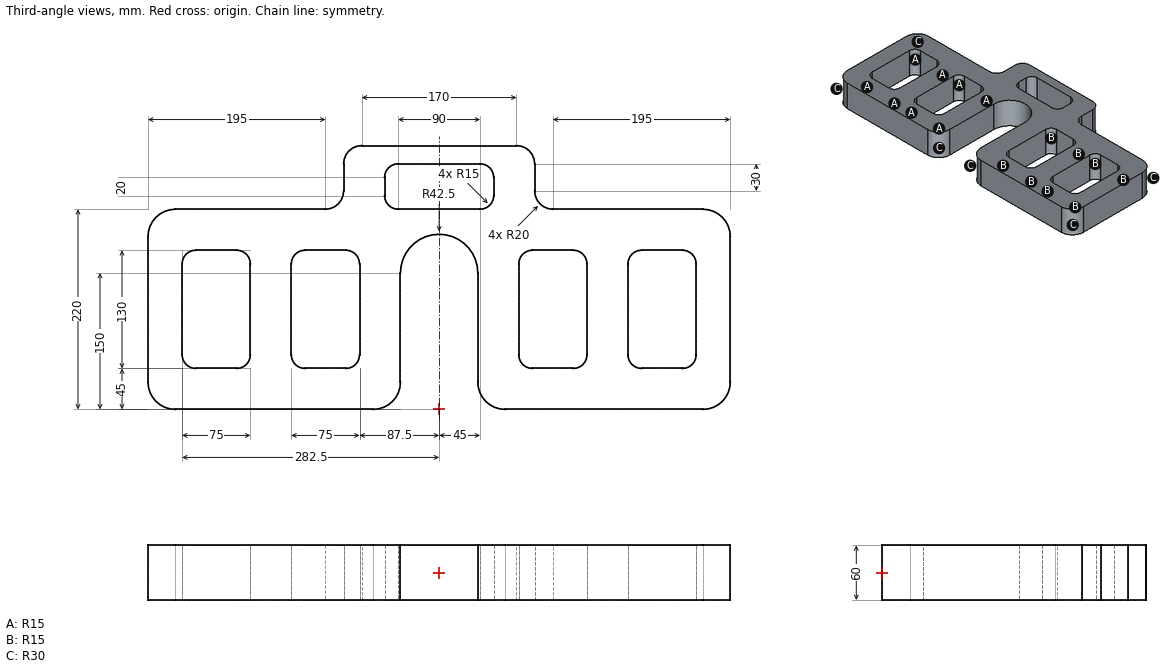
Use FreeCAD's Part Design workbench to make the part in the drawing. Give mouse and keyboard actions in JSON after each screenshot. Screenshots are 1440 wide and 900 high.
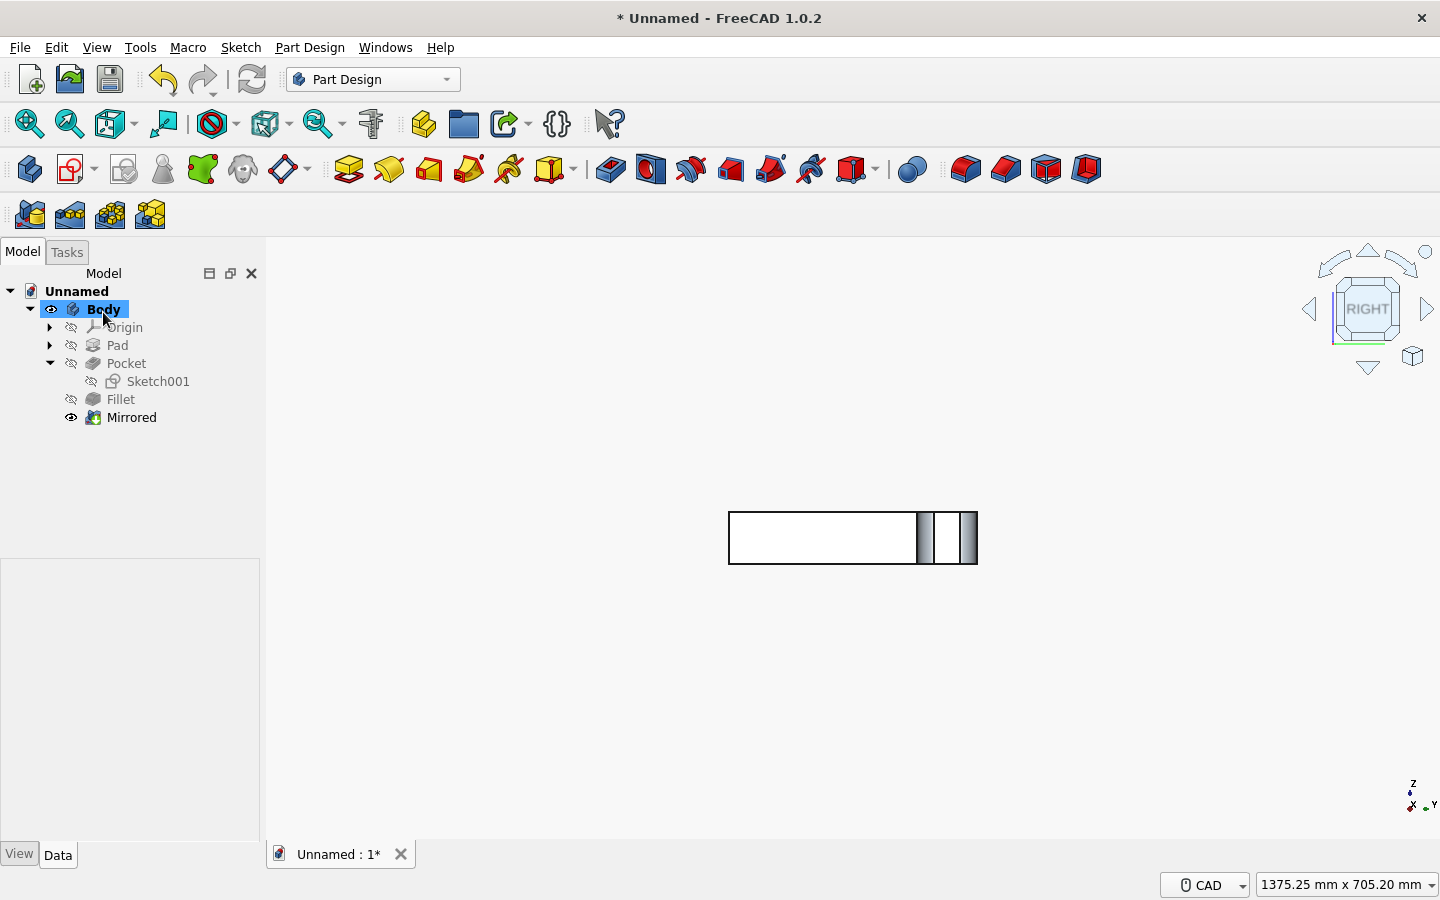
{"action": "key", "text": "5"}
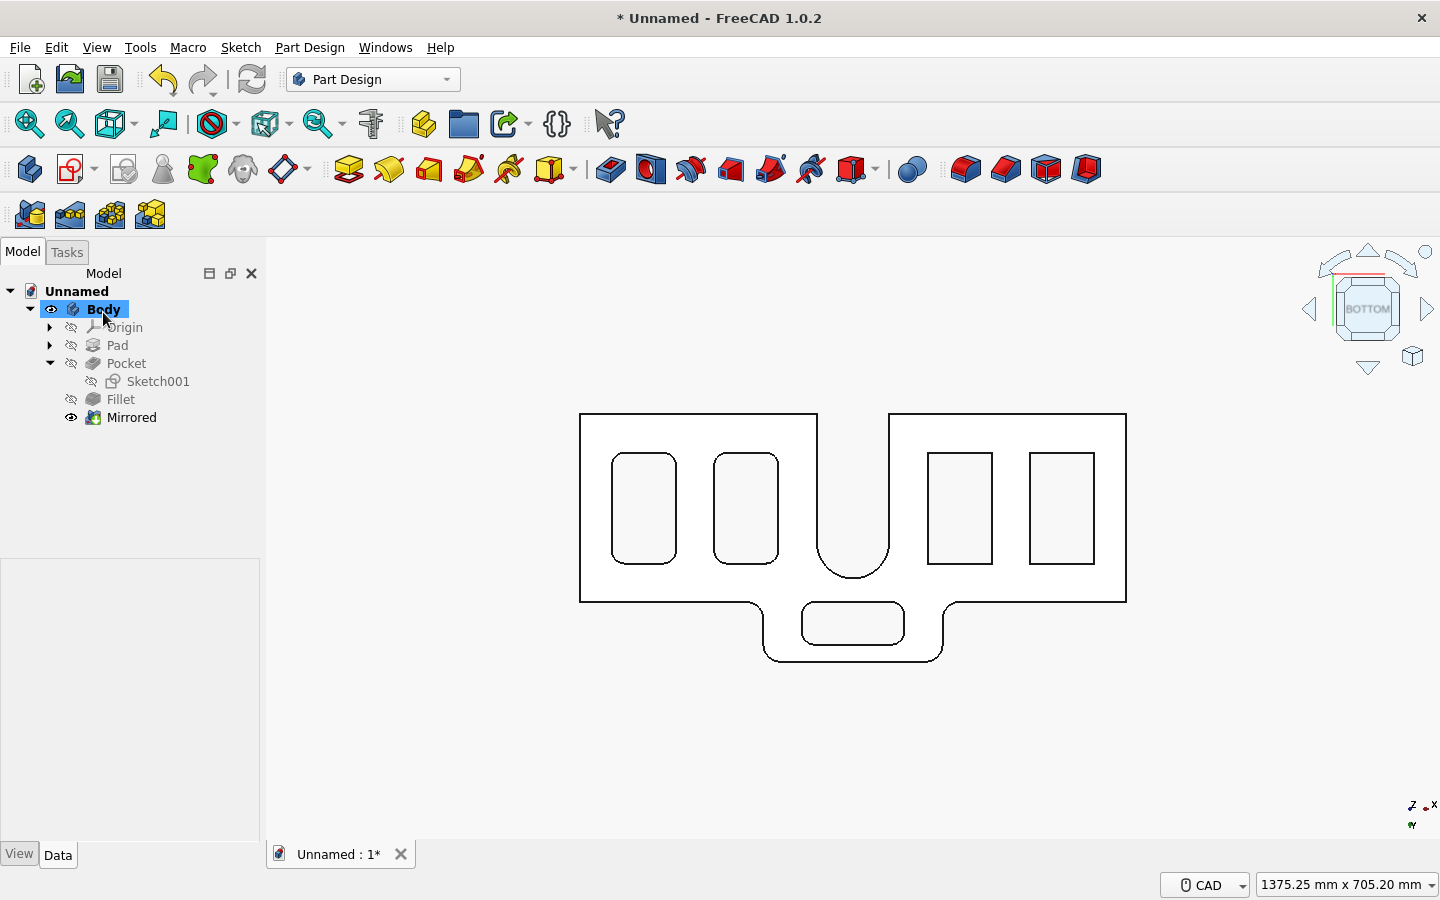
{"action": "key", "text": "4"}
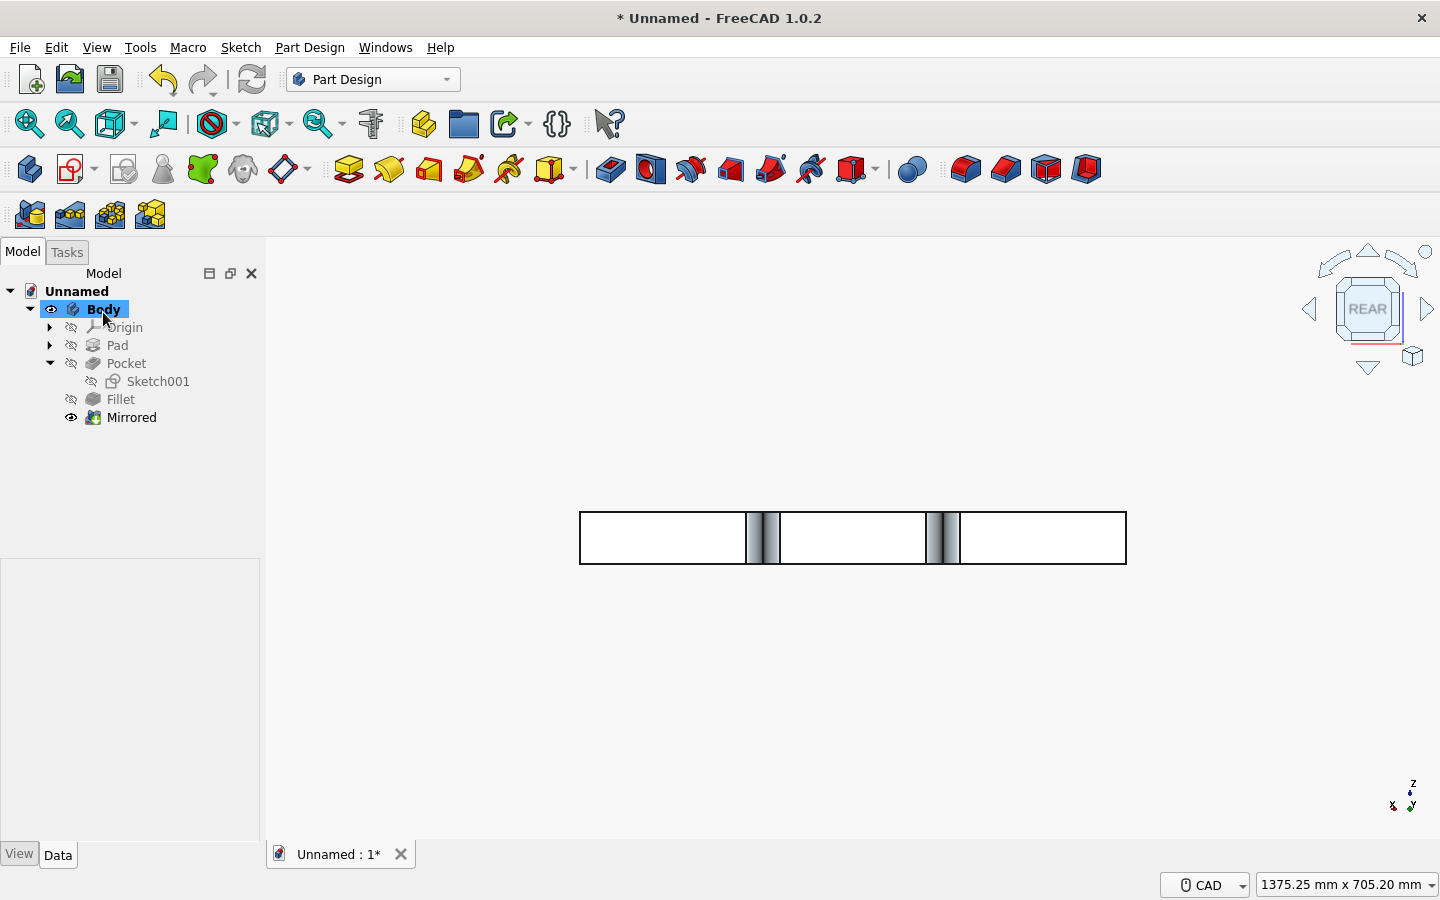
{"action": "key", "text": "6"}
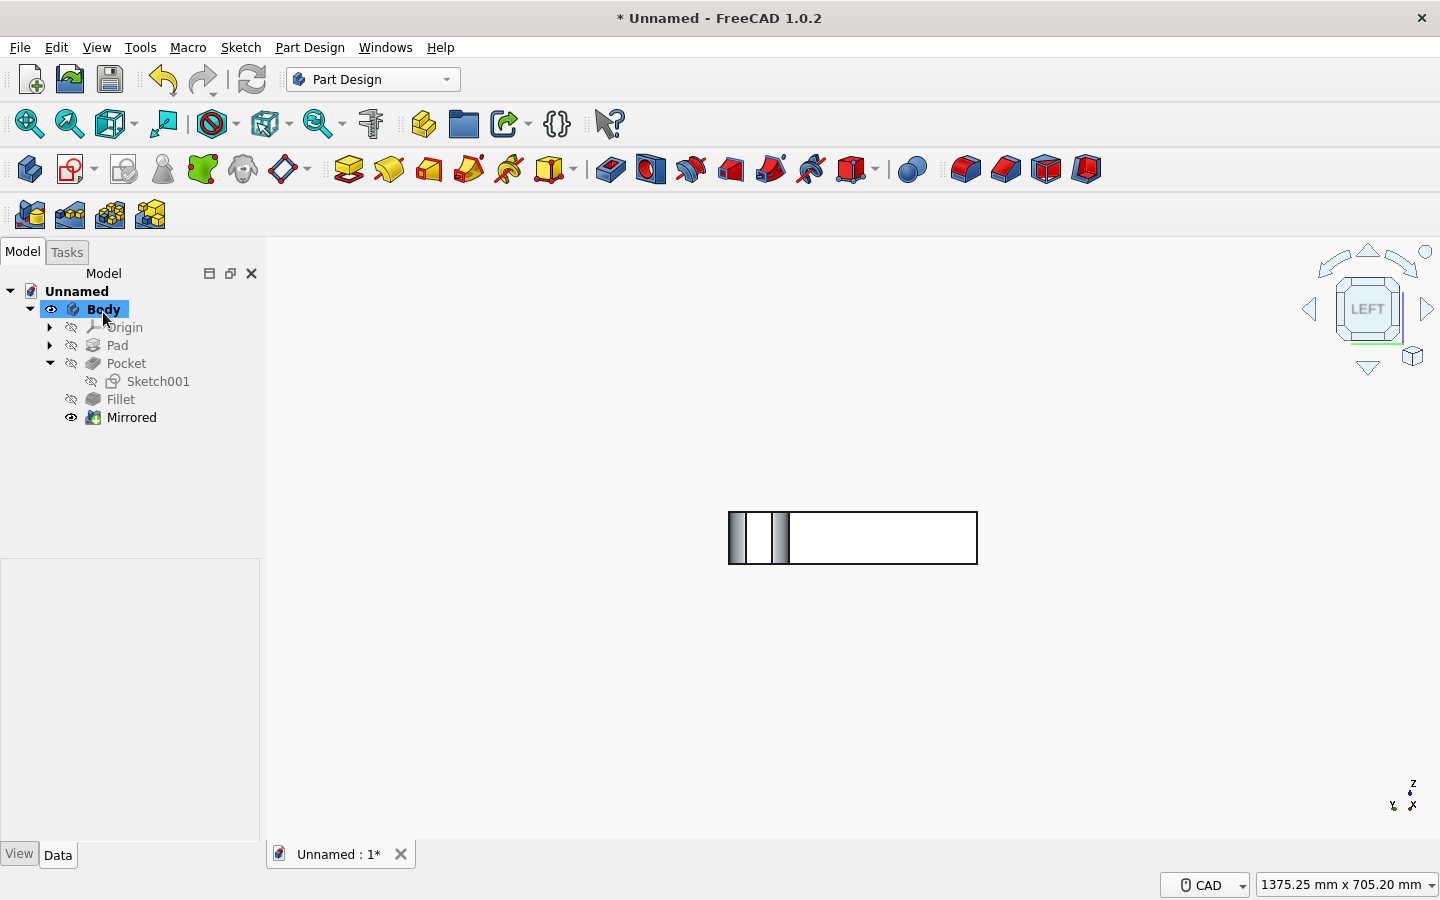
{"action": "left_click", "coordinate": [30, 124]}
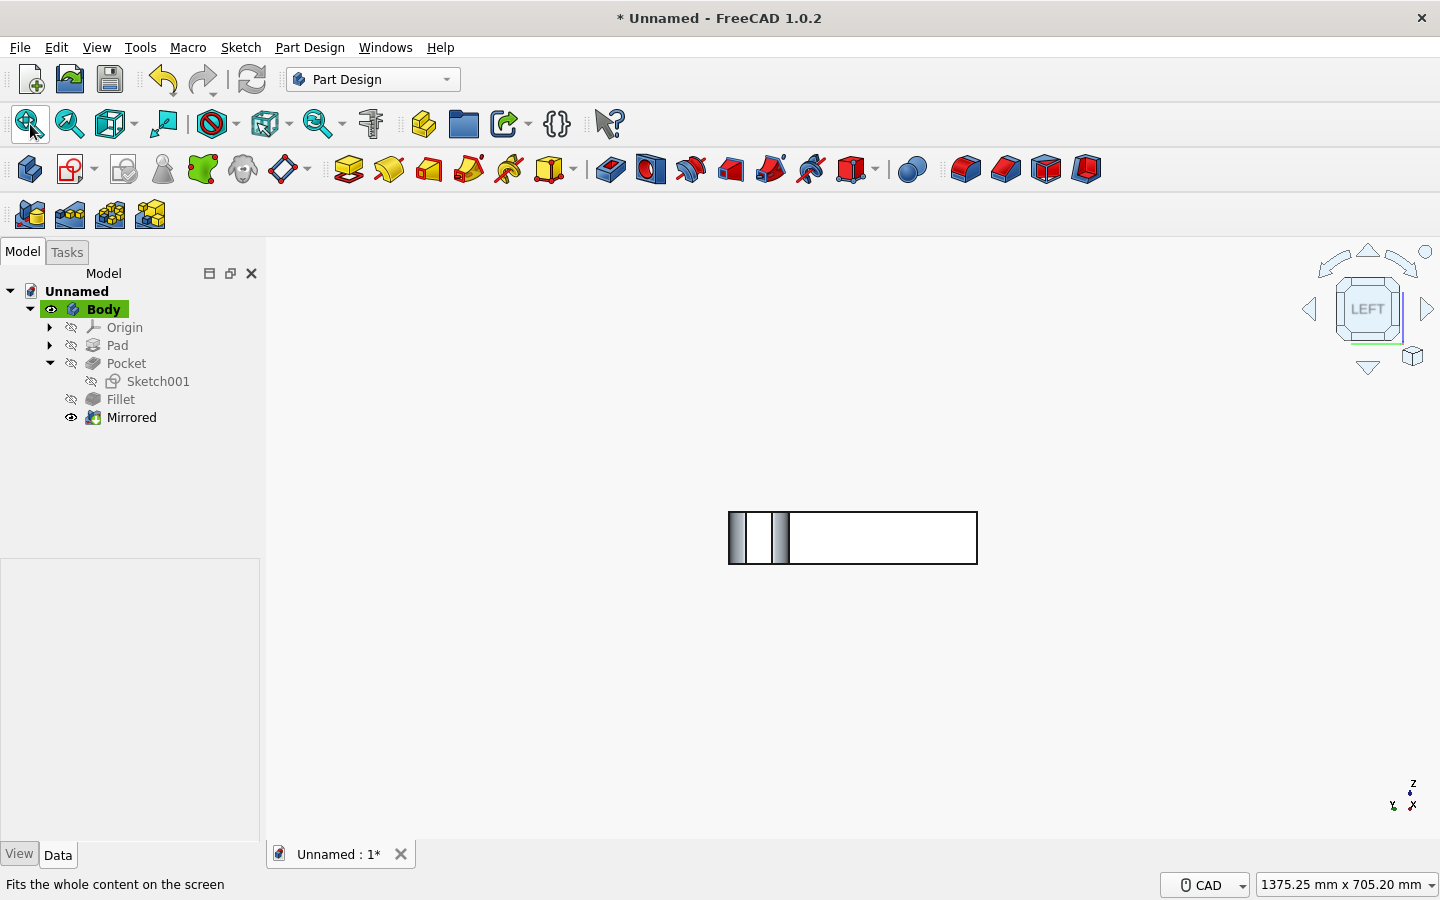
{"action": "key", "text": "v 3"}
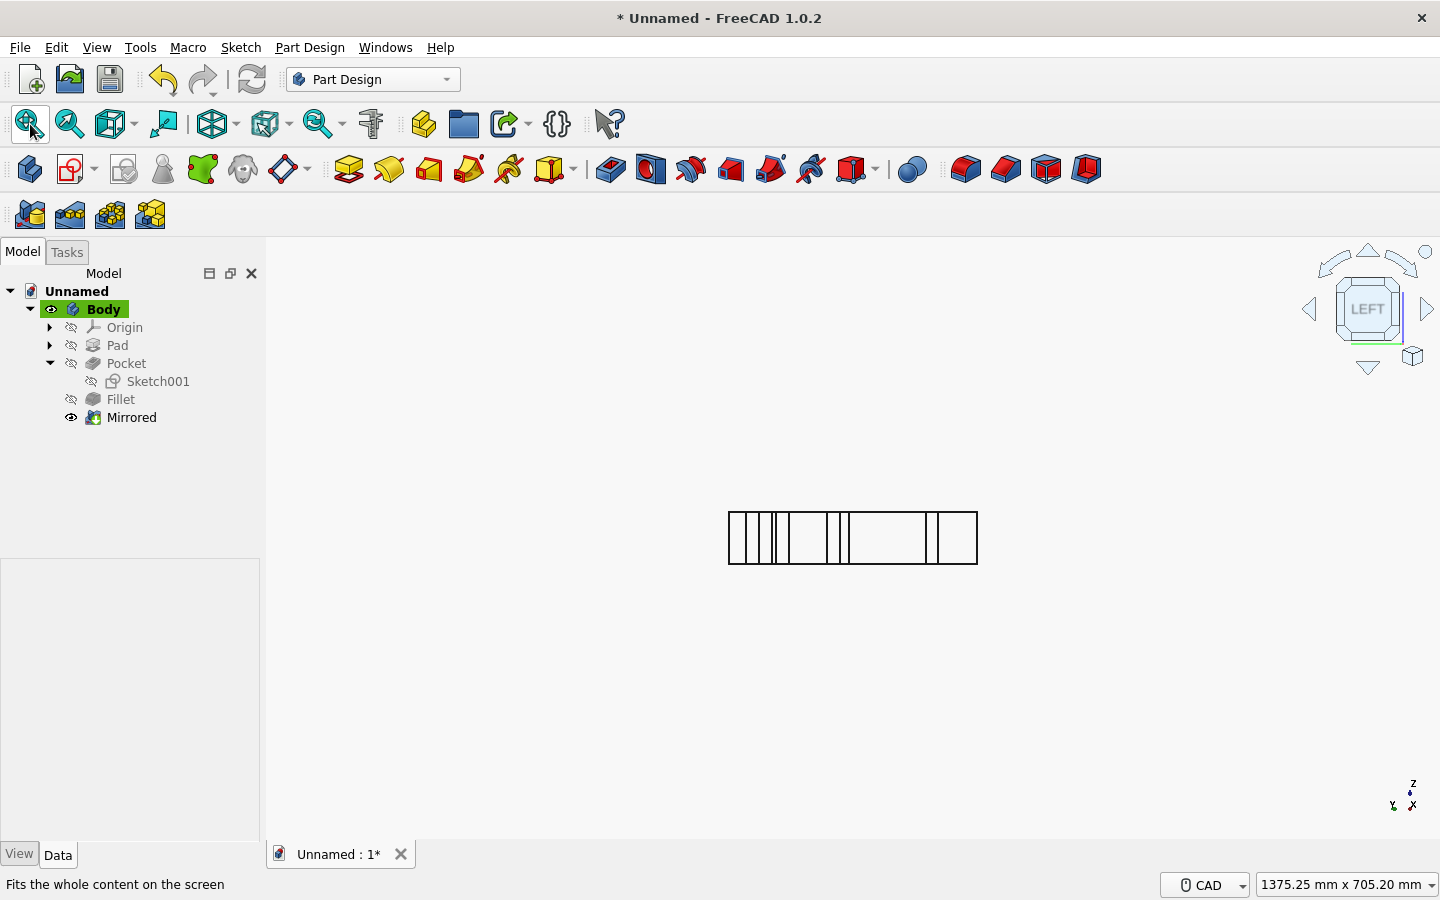
{"action": "key", "text": "0"}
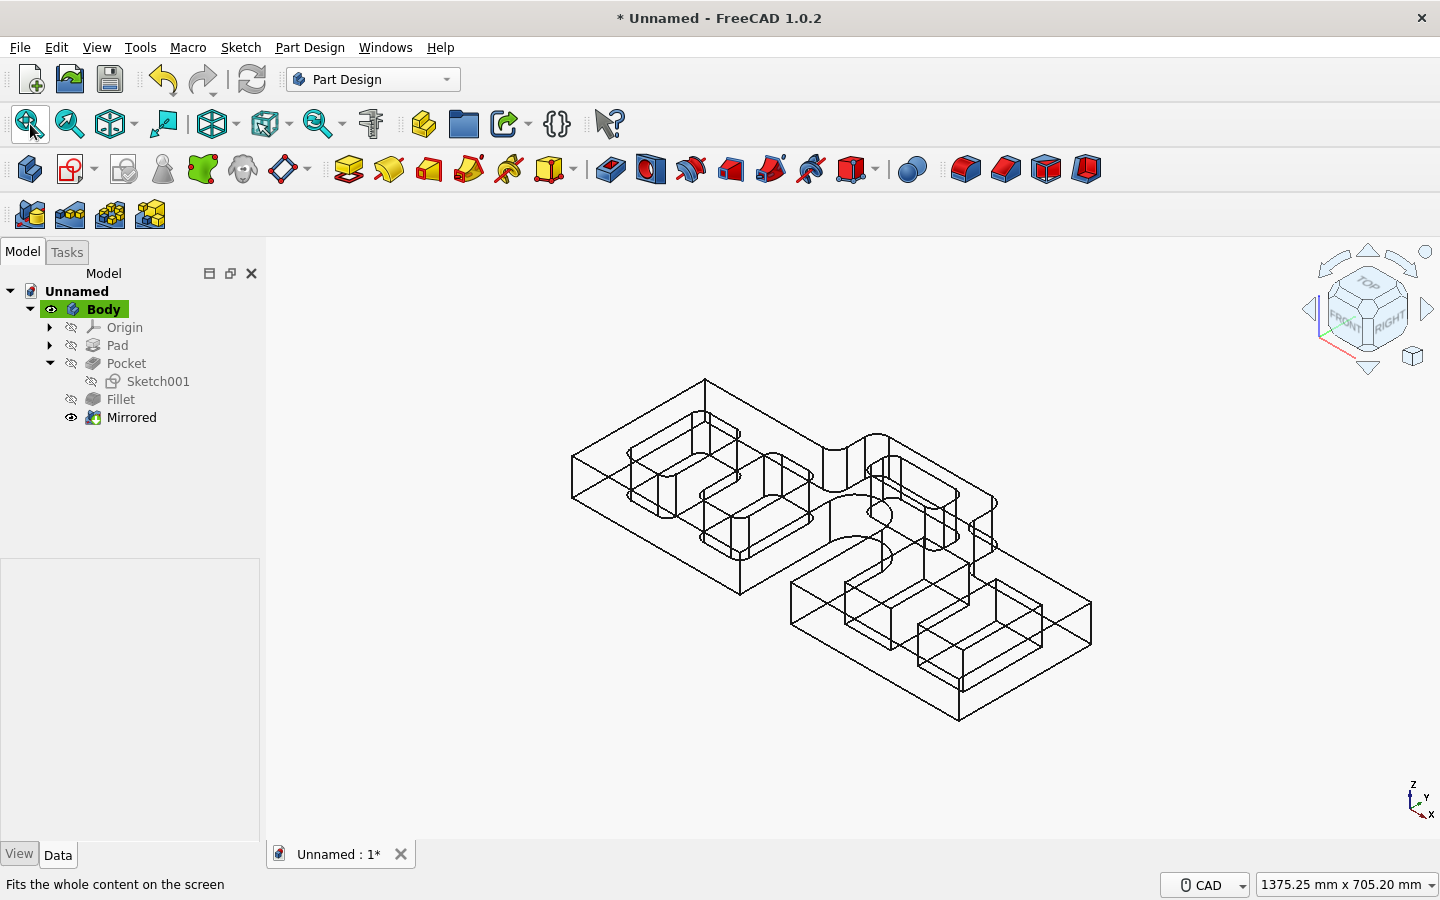
{"action": "left_click", "coordinate": [996, 599]}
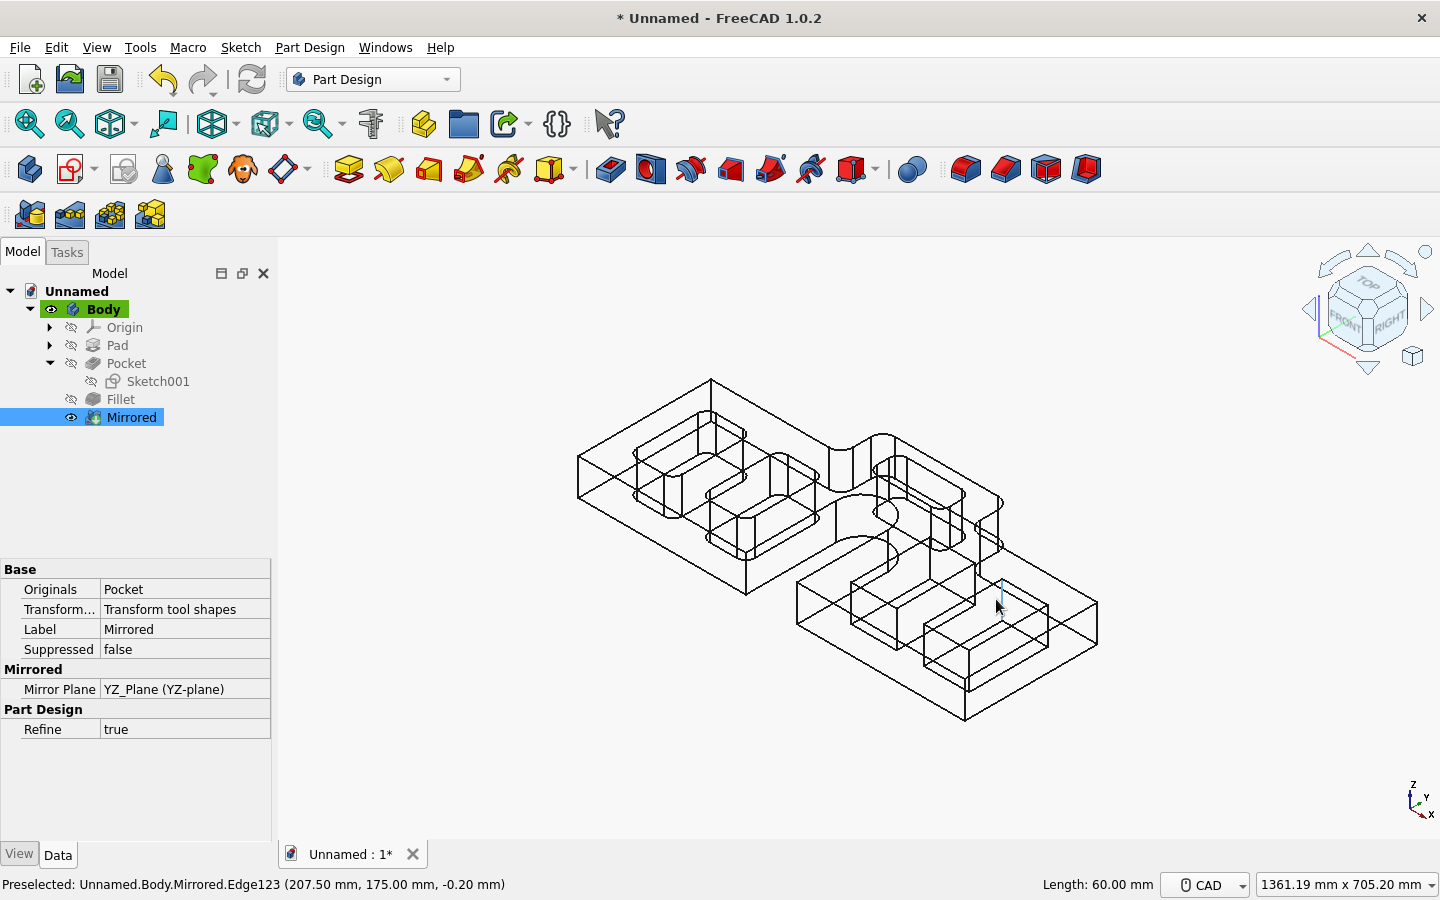
{"action": "left_click", "coordinate": [924, 644], "text": "ctrl"}